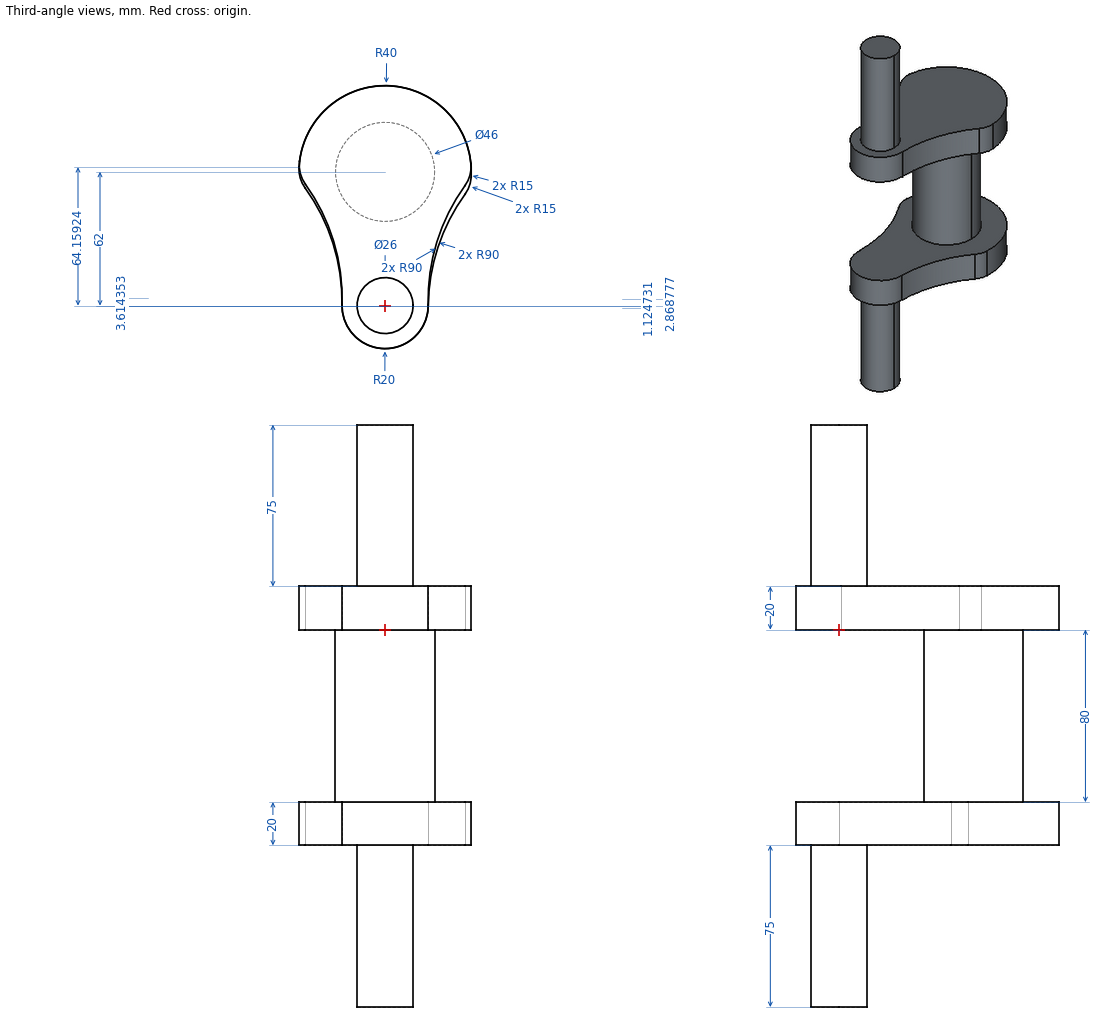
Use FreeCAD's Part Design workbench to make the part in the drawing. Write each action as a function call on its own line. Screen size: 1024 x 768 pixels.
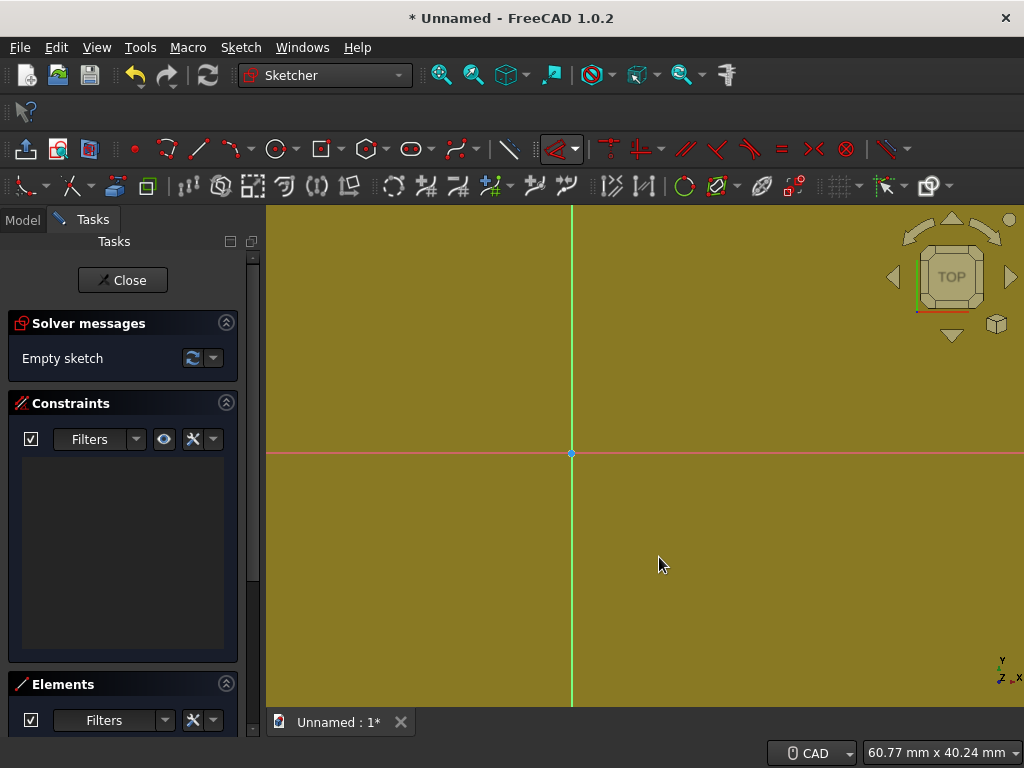
click(276, 150)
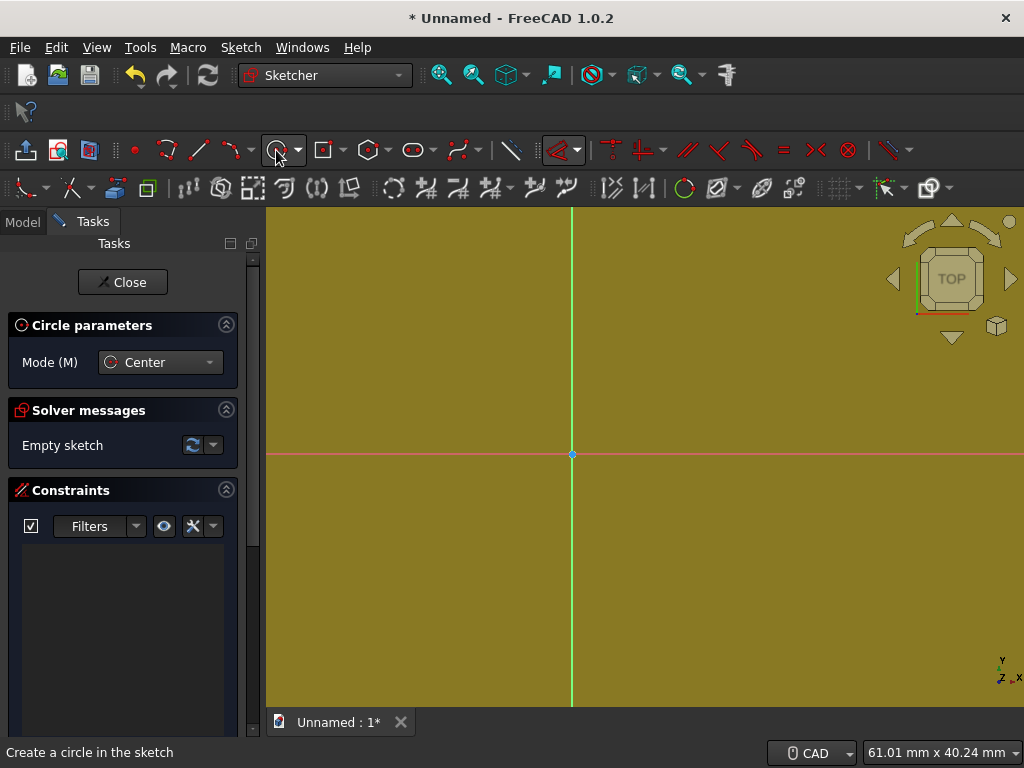
click(572, 454)
move(686, 340)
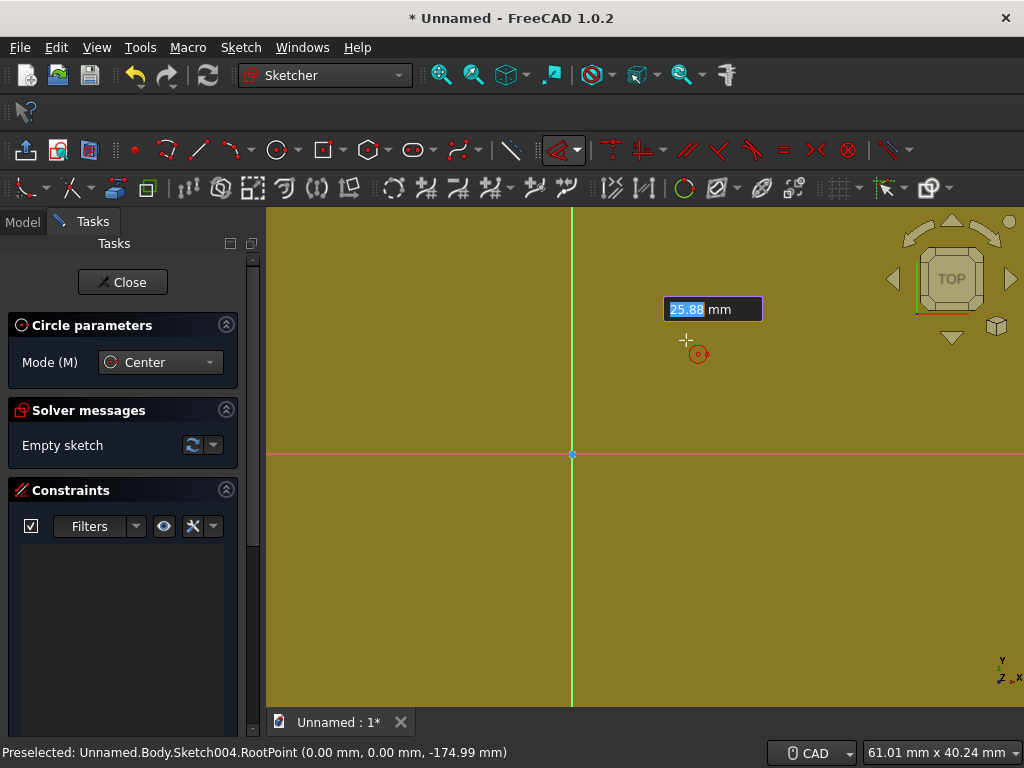
text(26)
key(Return)
key(Escape)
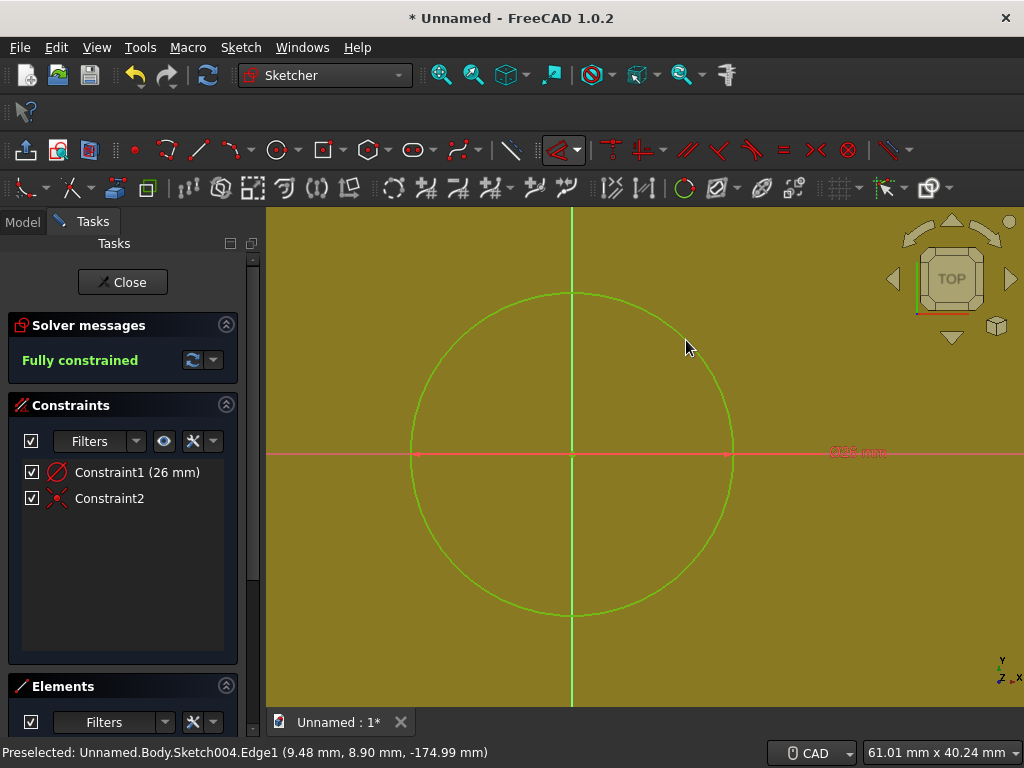
click(123, 282)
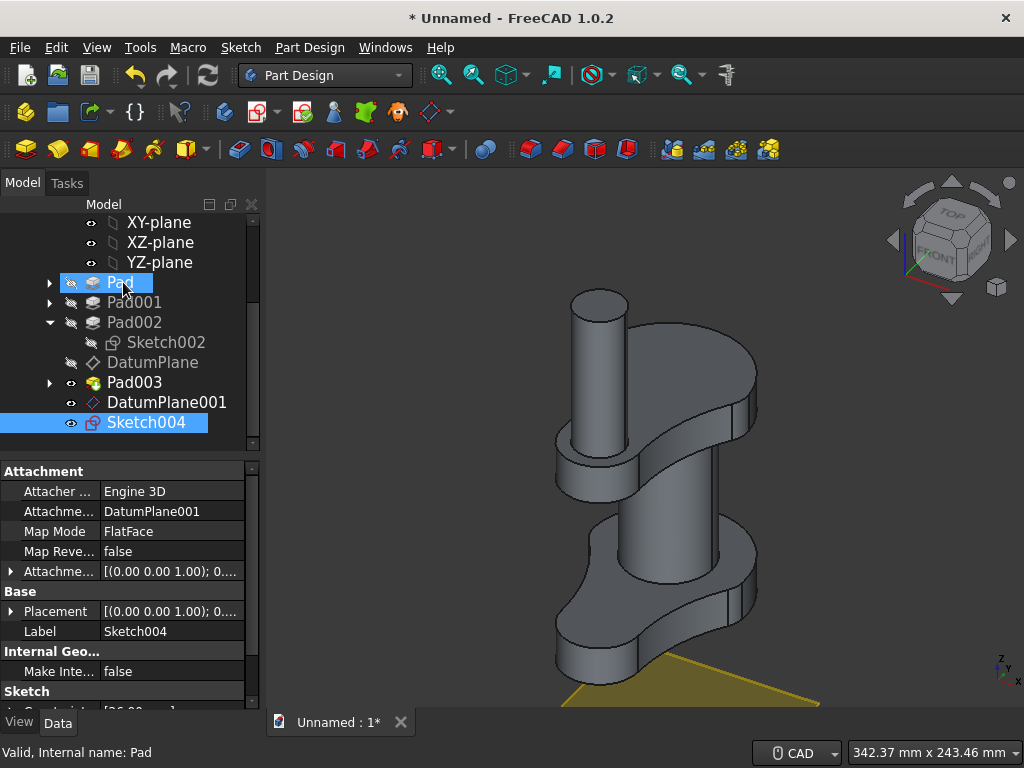
click(26, 150)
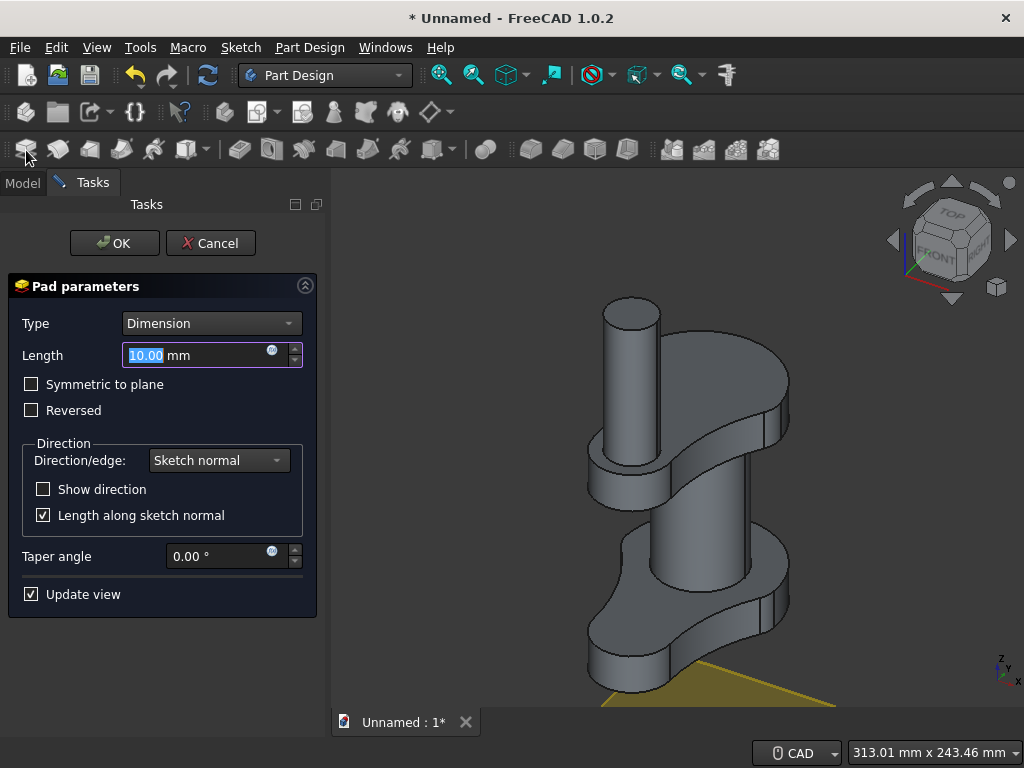
text(75)
key(Tab)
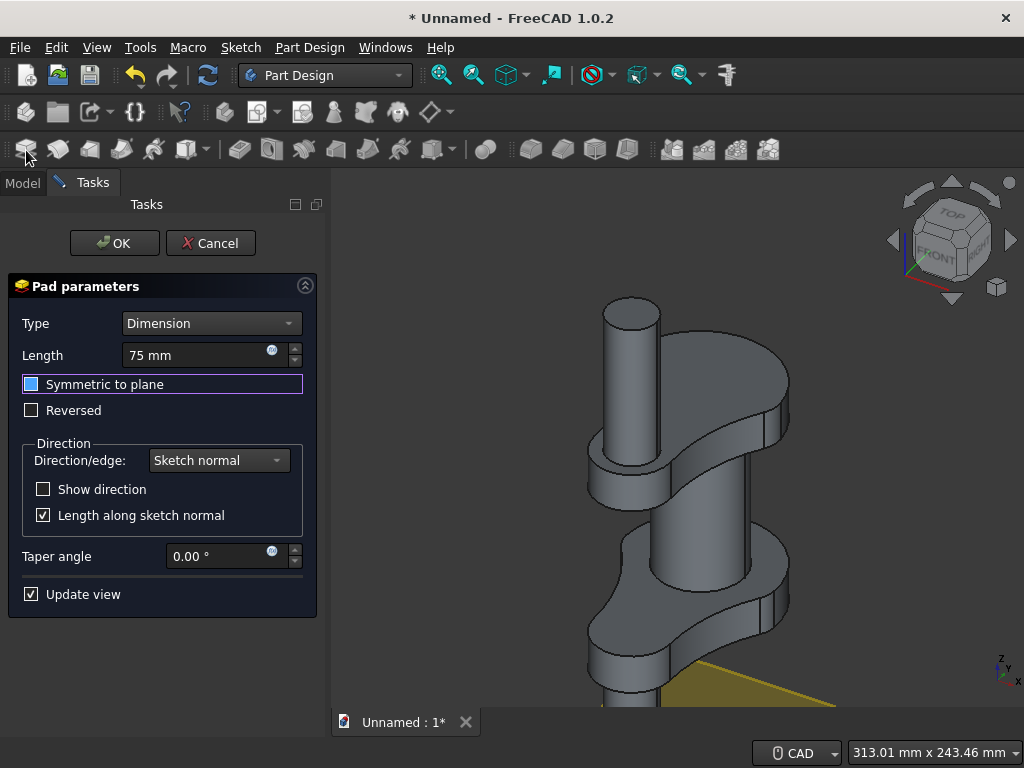
click(115, 243)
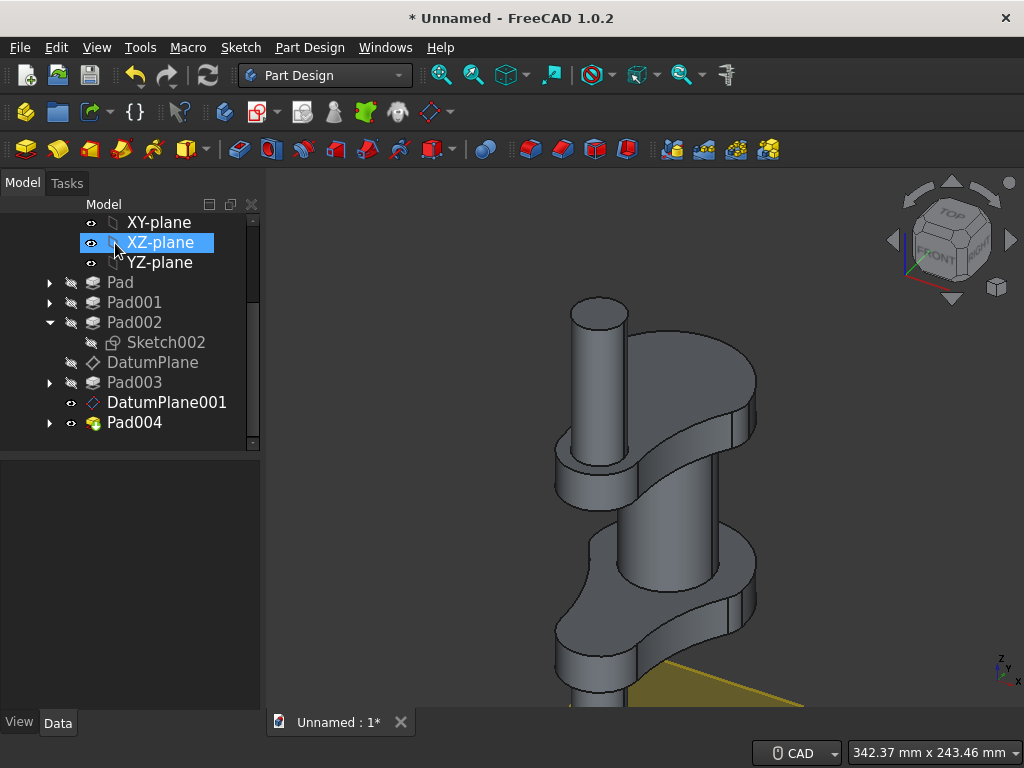
click(116, 403)
key(space)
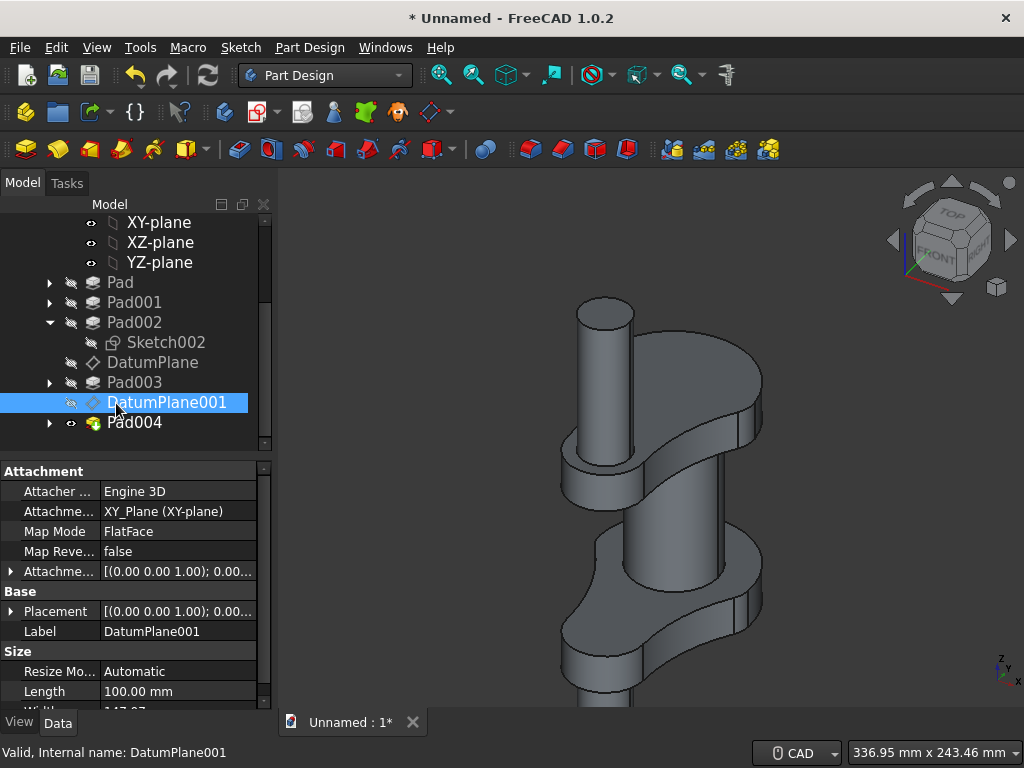
key(0)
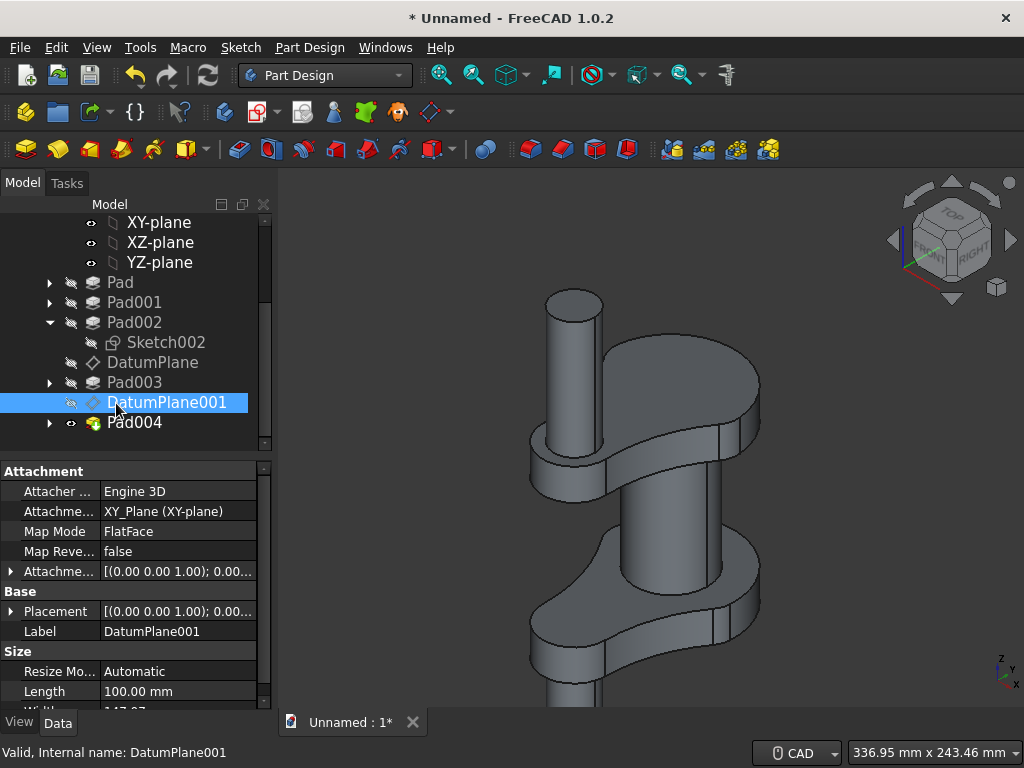
click(442, 76)